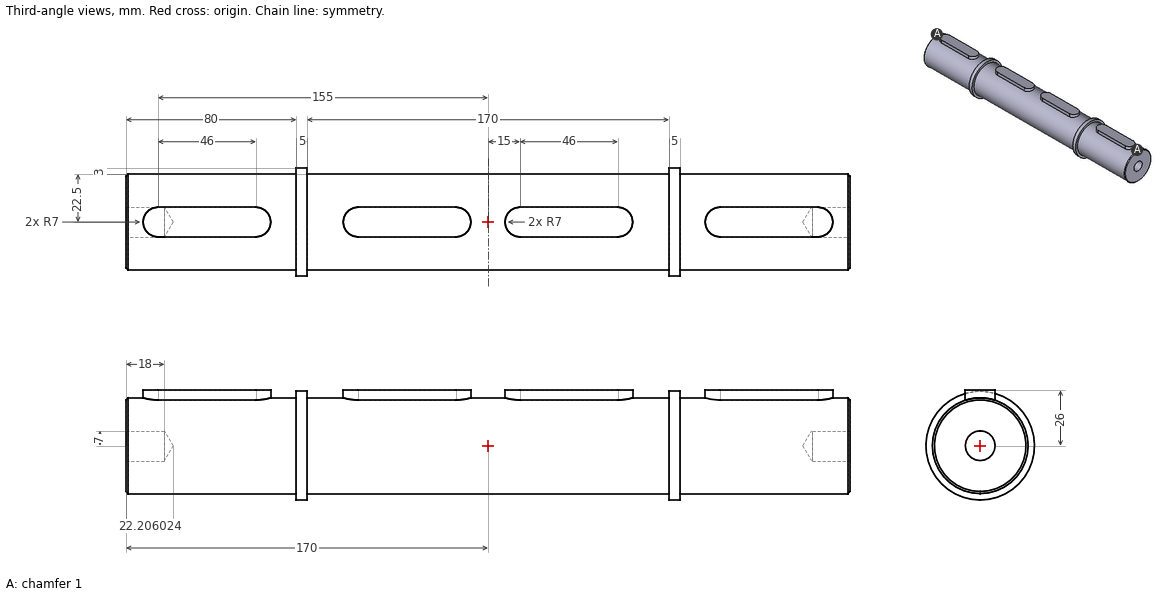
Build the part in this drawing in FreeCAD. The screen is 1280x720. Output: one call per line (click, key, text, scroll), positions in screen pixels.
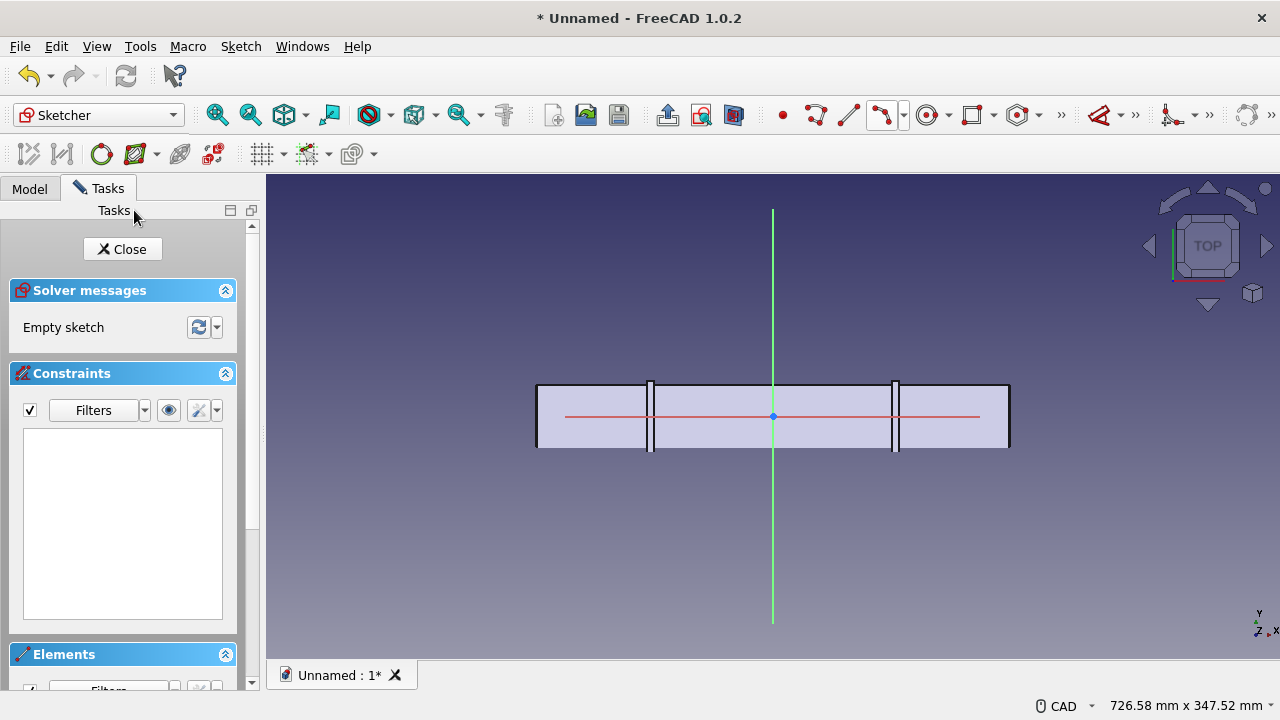
scroll(571, 416, up, 10)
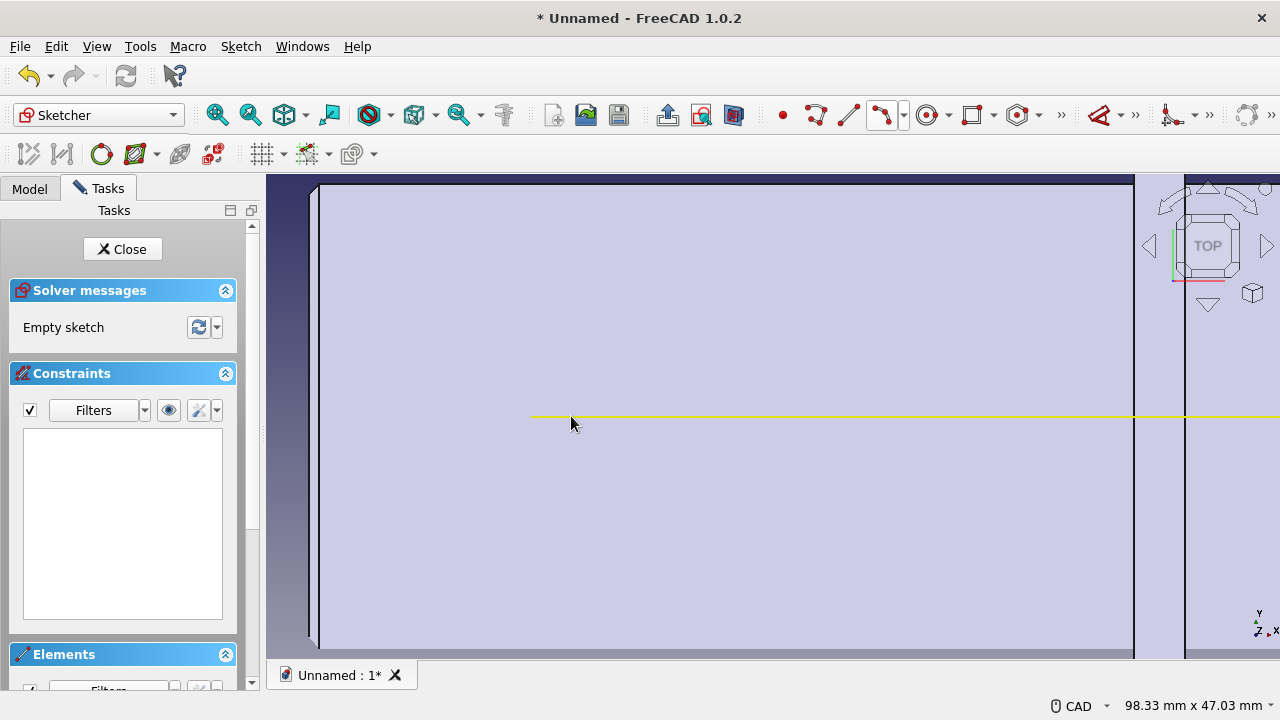
key(g)
key(s)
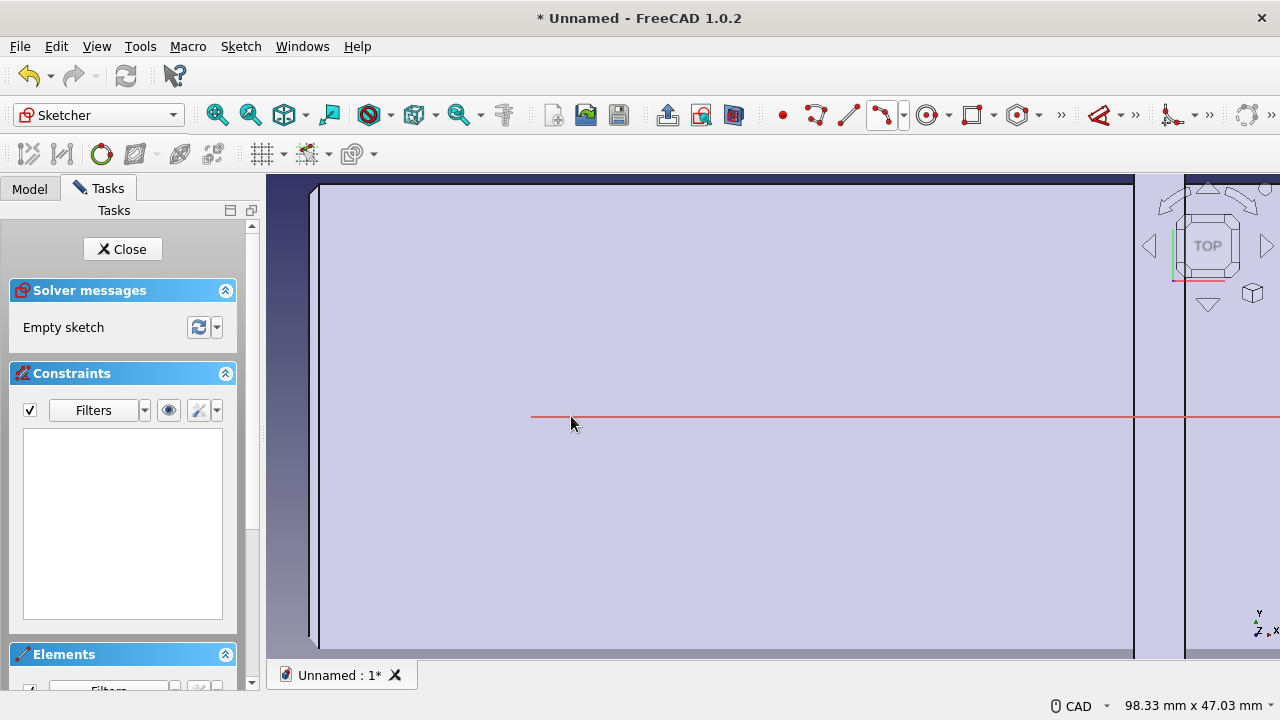
click(463, 416)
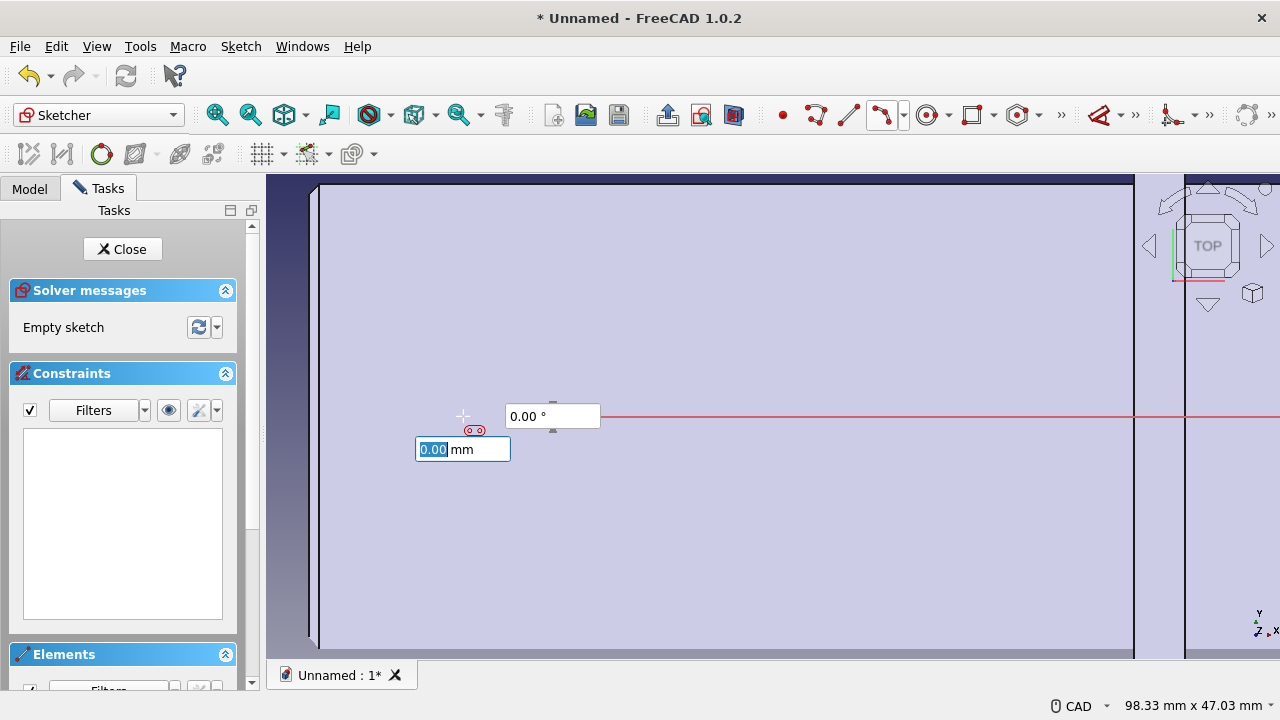
click(938, 408)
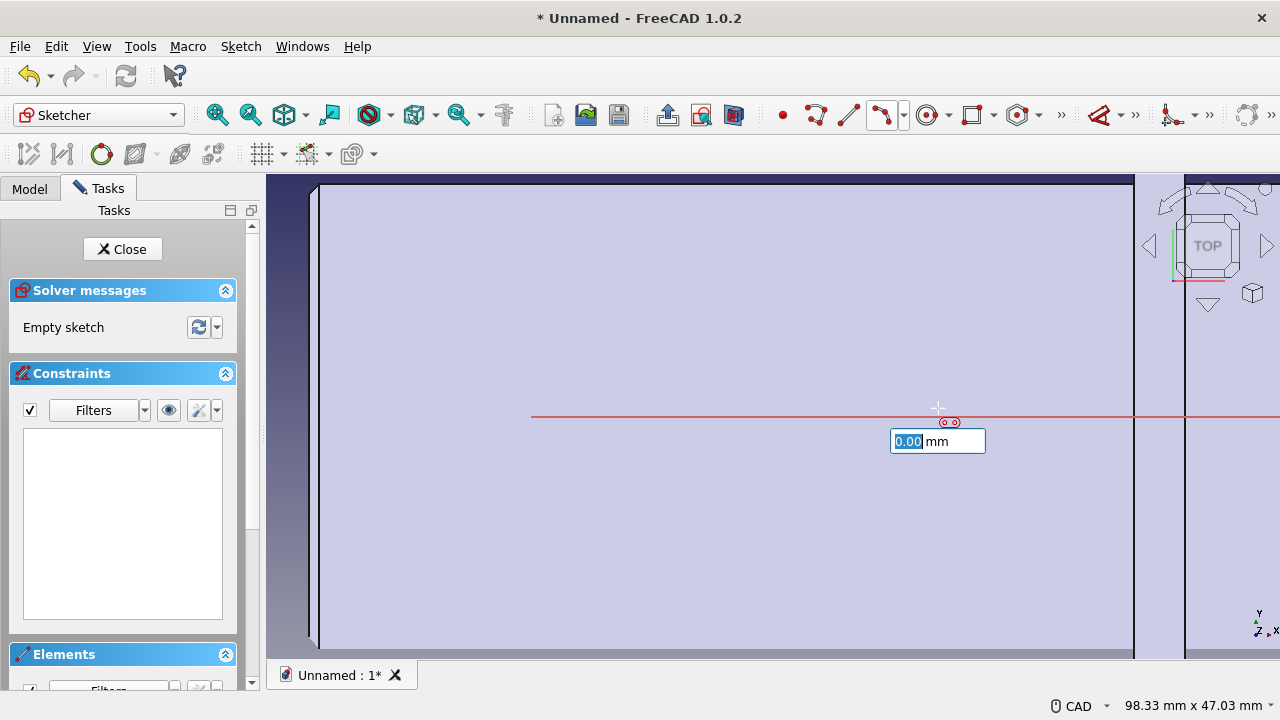
click(700, 344)
key(Escape)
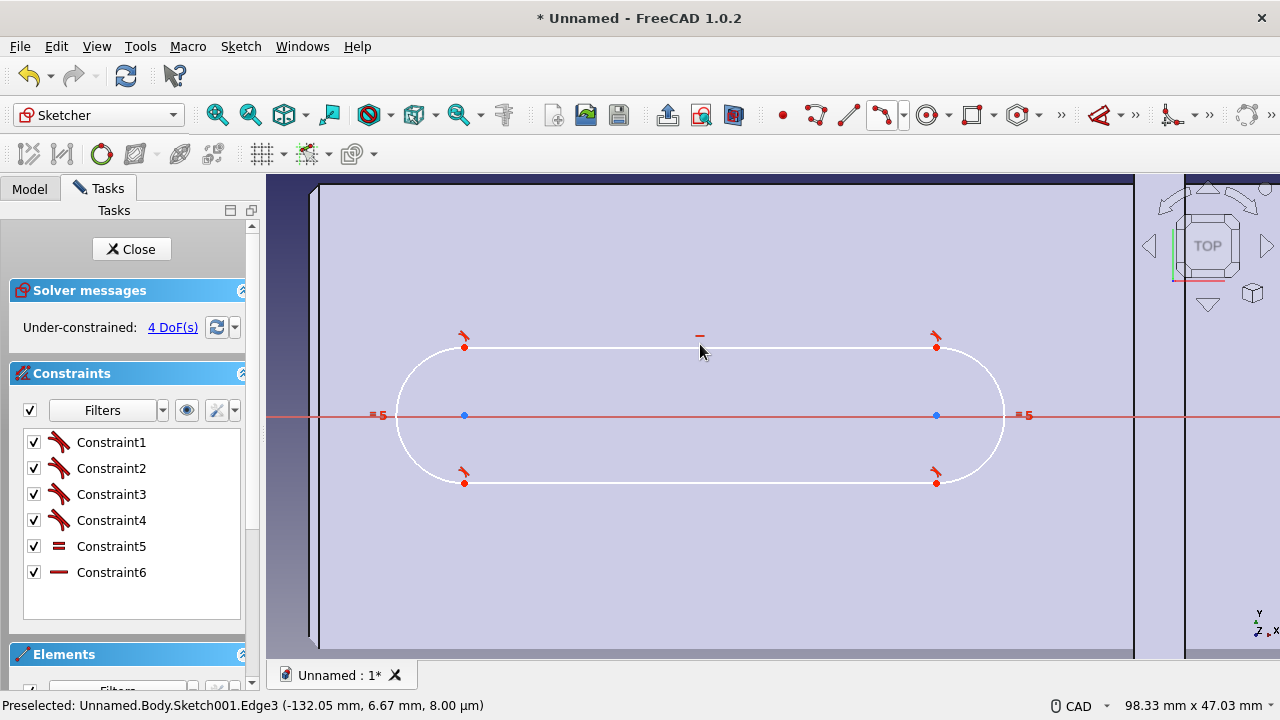
click(464, 415)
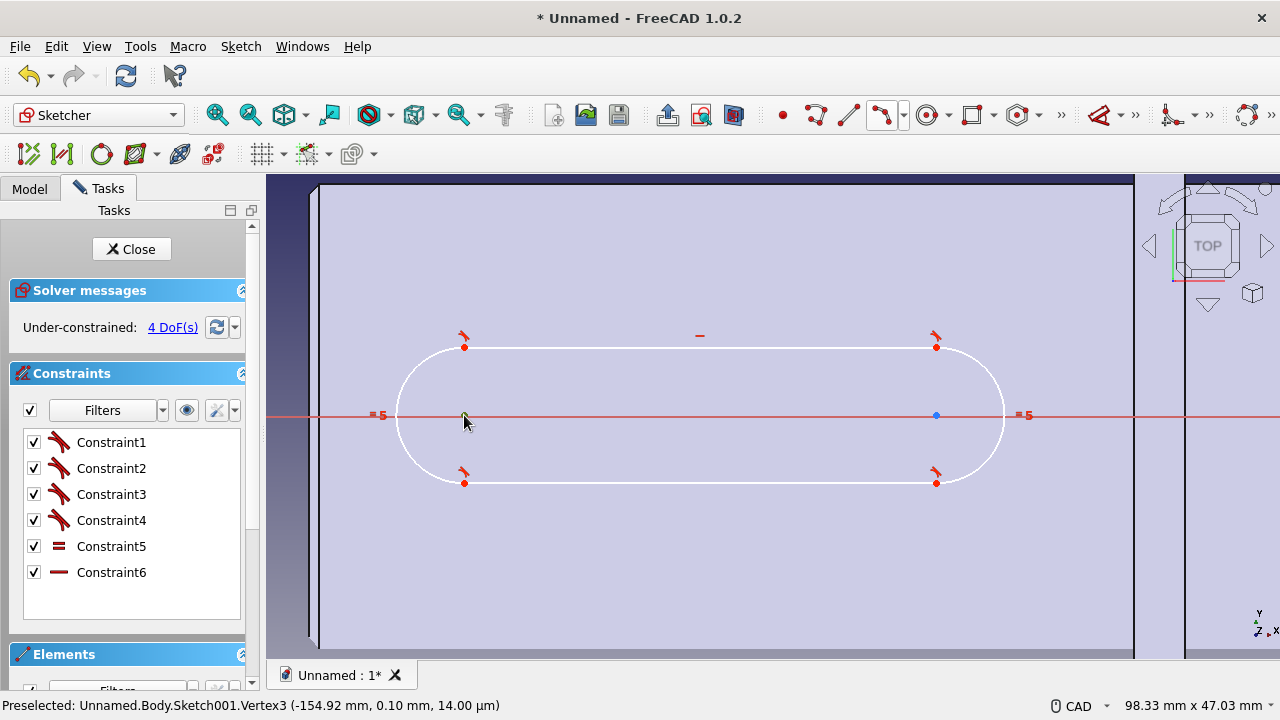
click(353, 416)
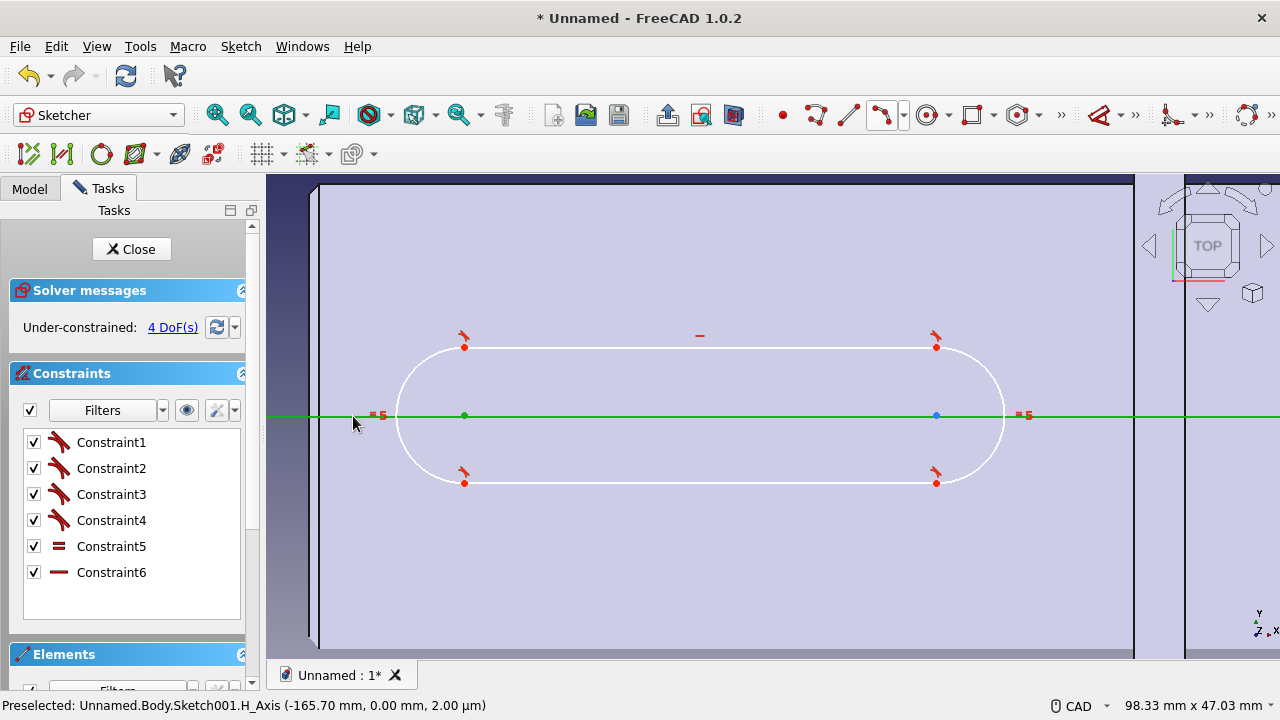
key(c)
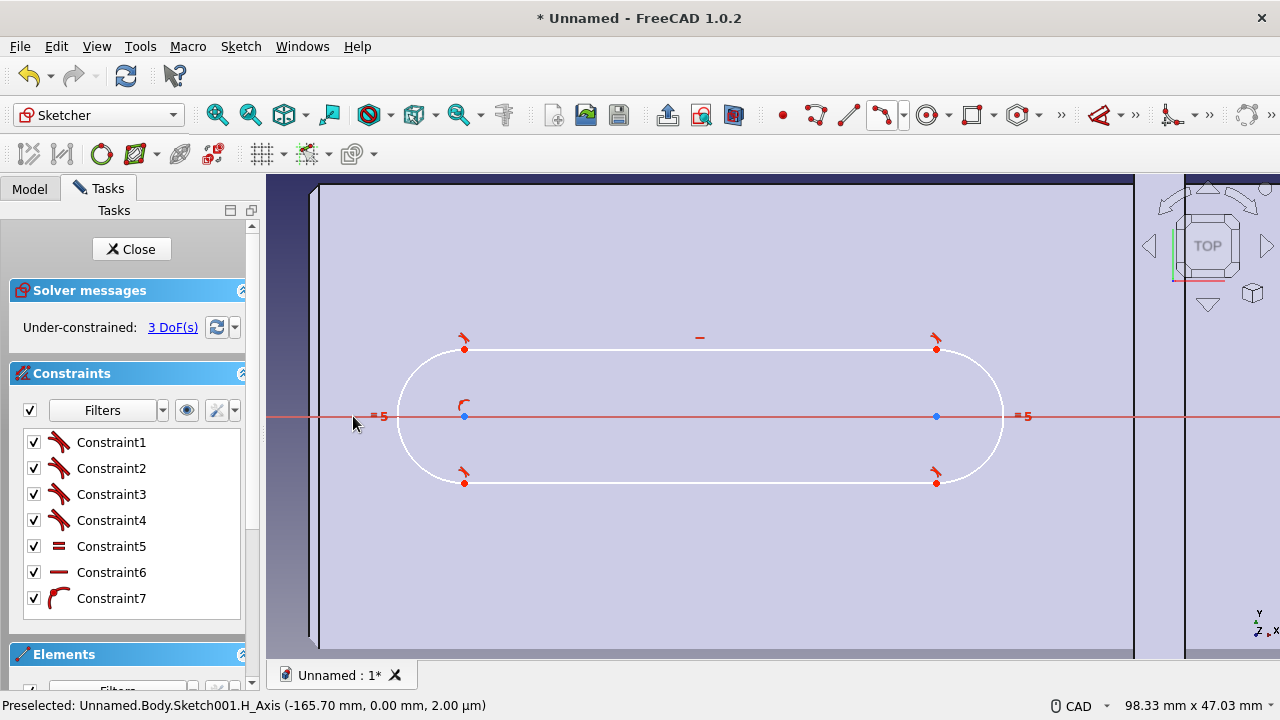
key(d)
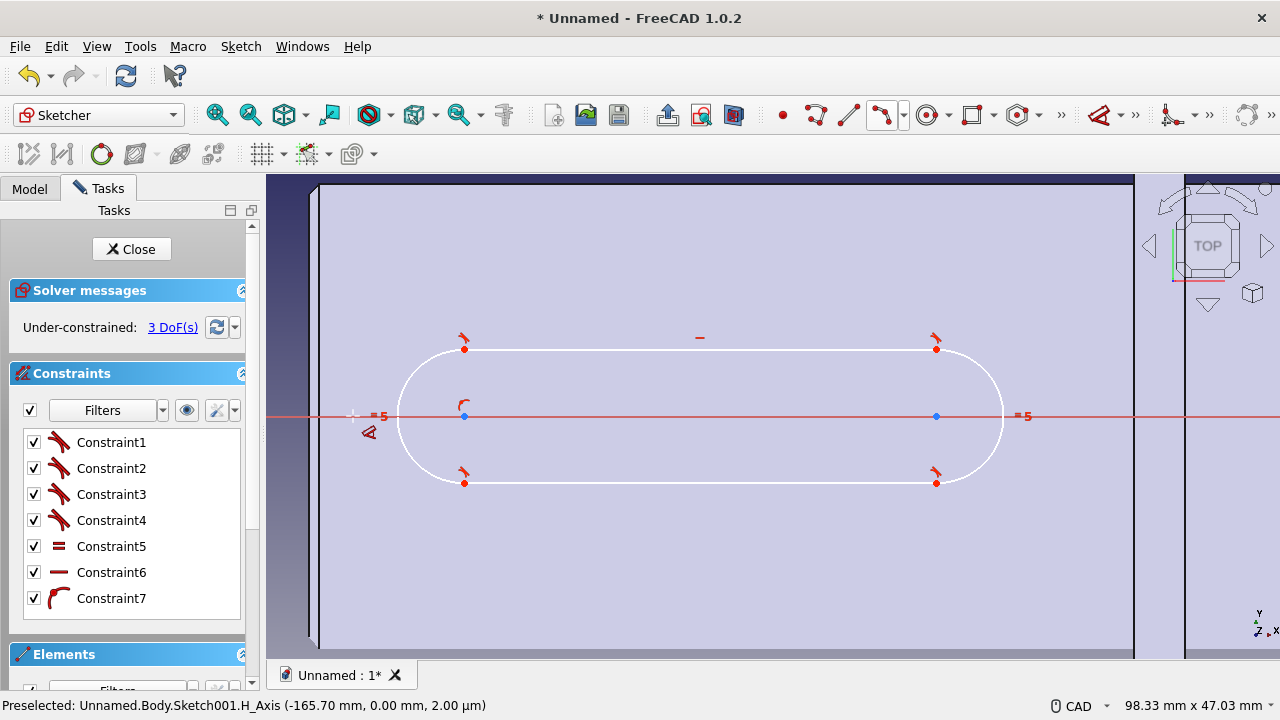
click(410, 377)
click(384, 358)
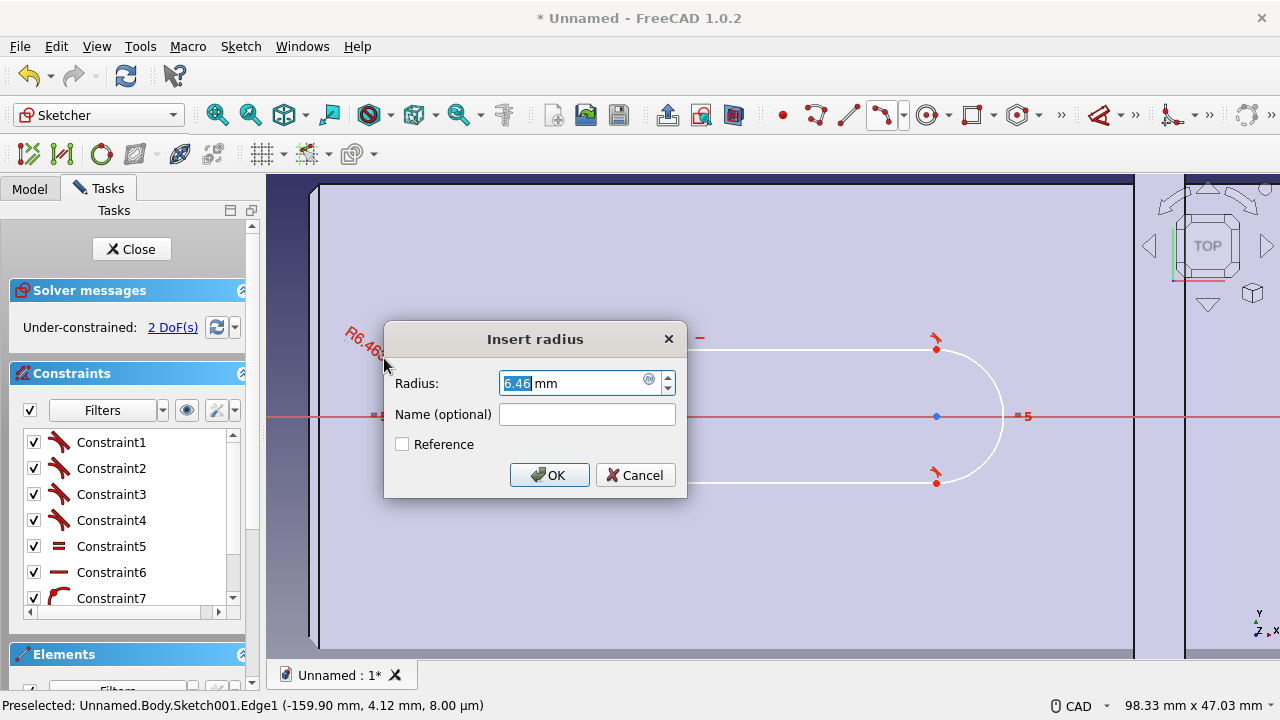
text(7)
key(Return)